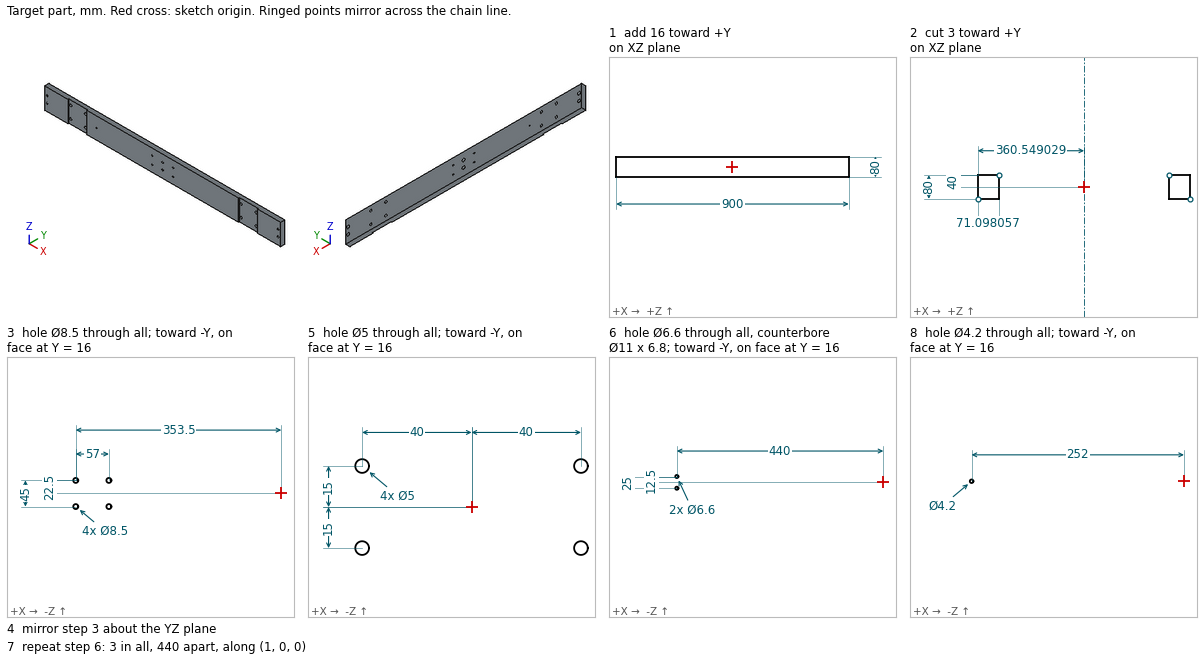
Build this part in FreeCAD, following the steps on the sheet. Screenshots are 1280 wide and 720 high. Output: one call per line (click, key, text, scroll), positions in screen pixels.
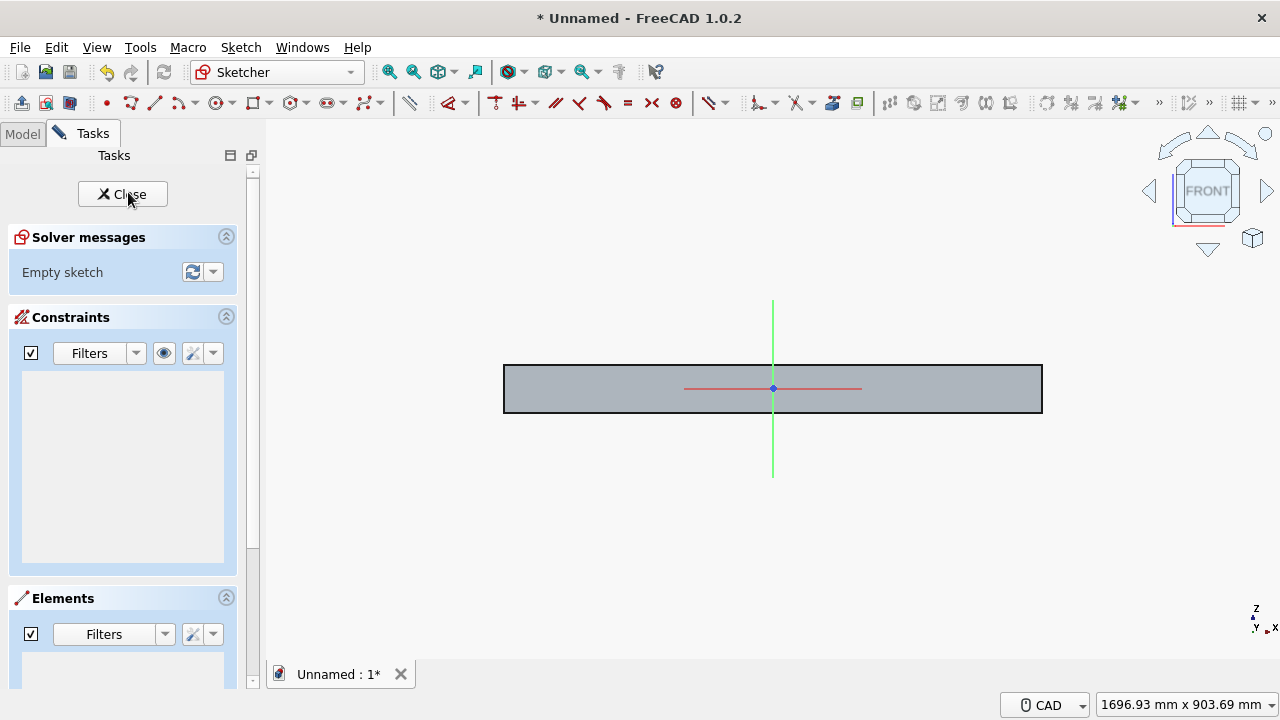
click(254, 104)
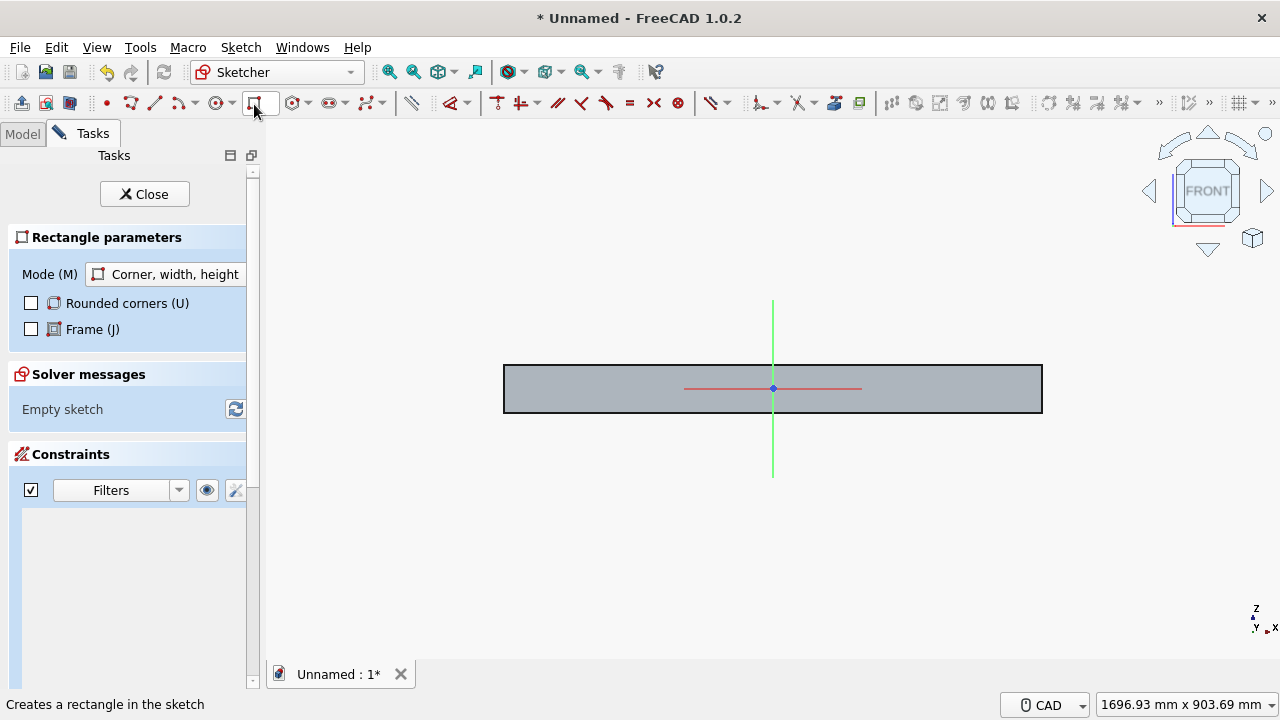
click(558, 365)
click(600, 413)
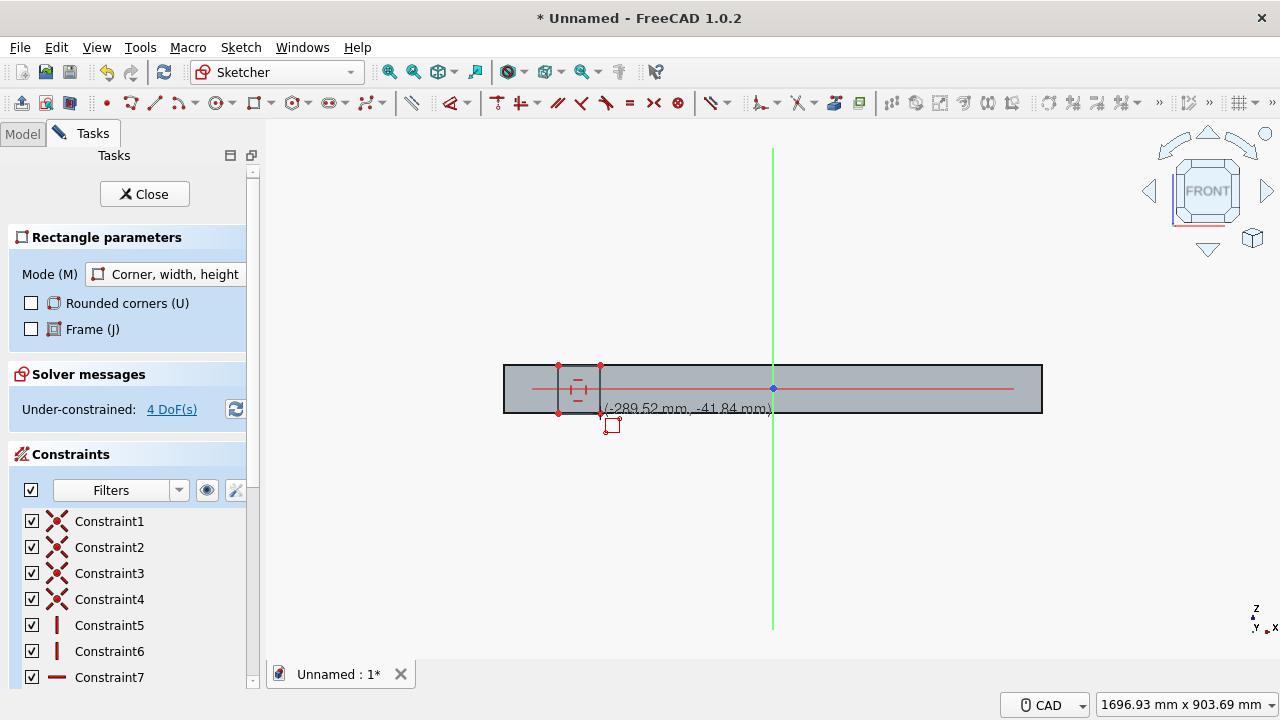
click(946, 365)
click(988, 413)
key(Escape)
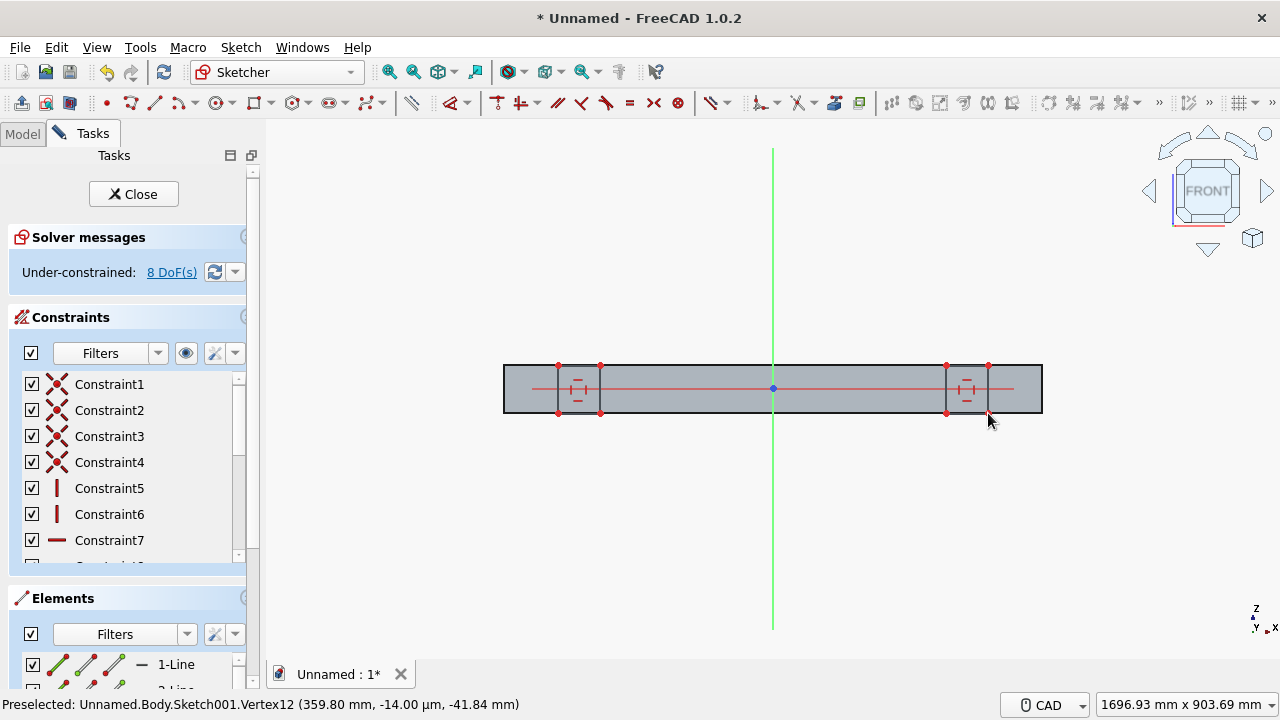
click(600, 366)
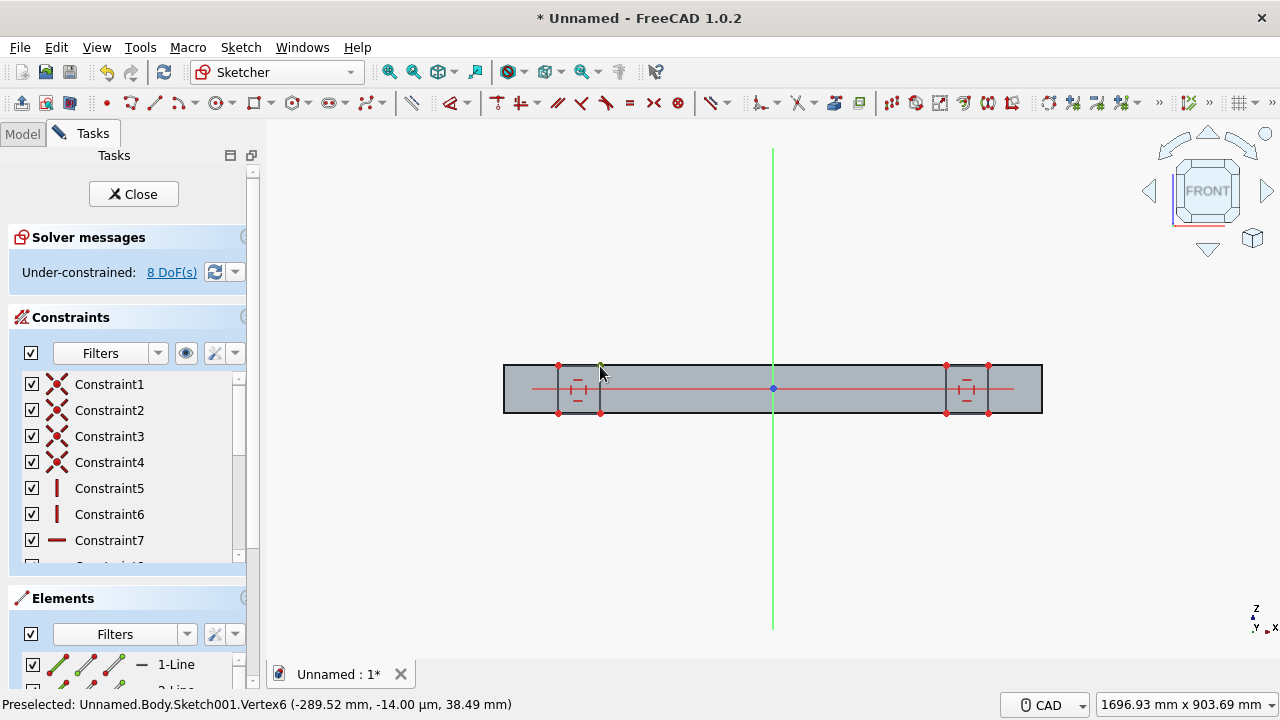
click(946, 366)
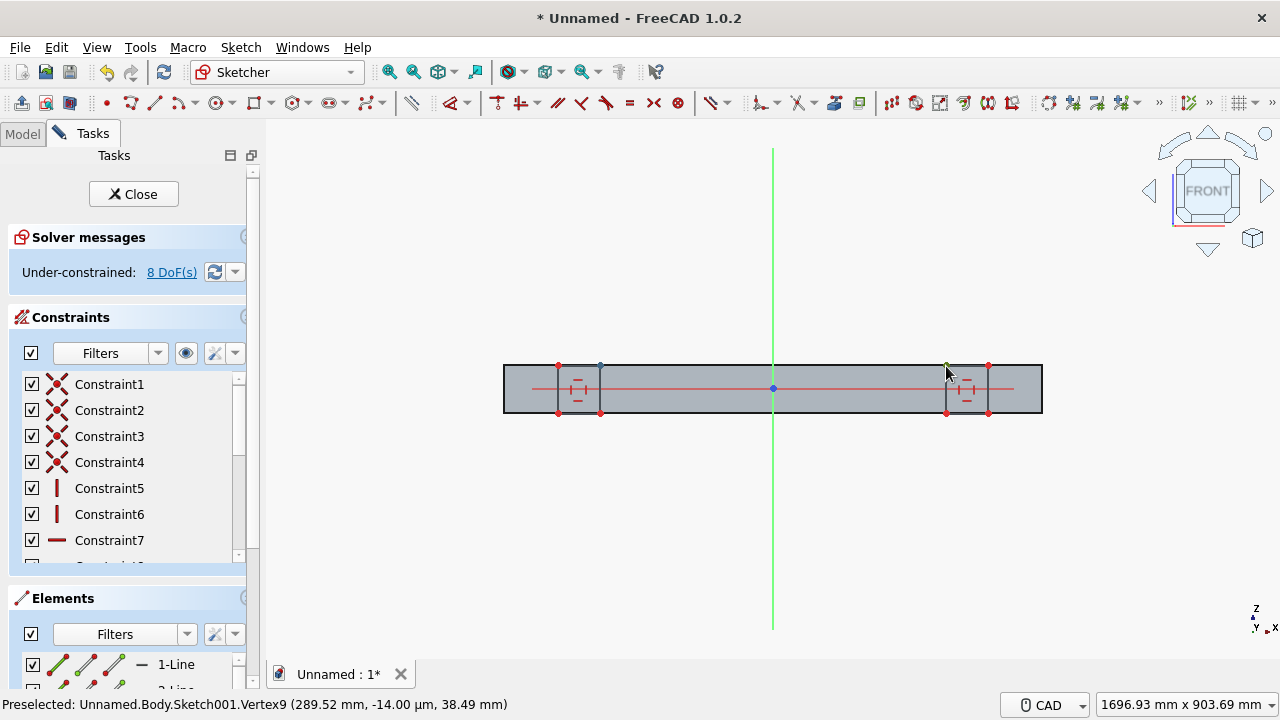
click(773, 596)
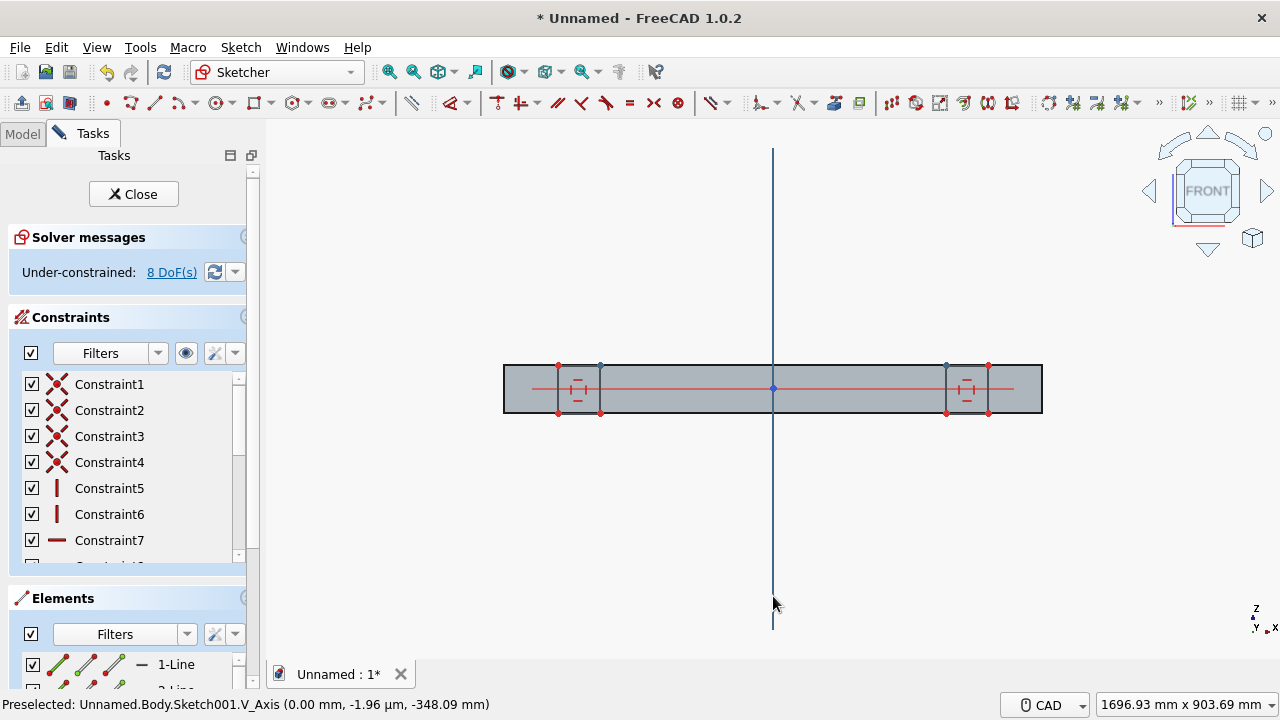
click(654, 104)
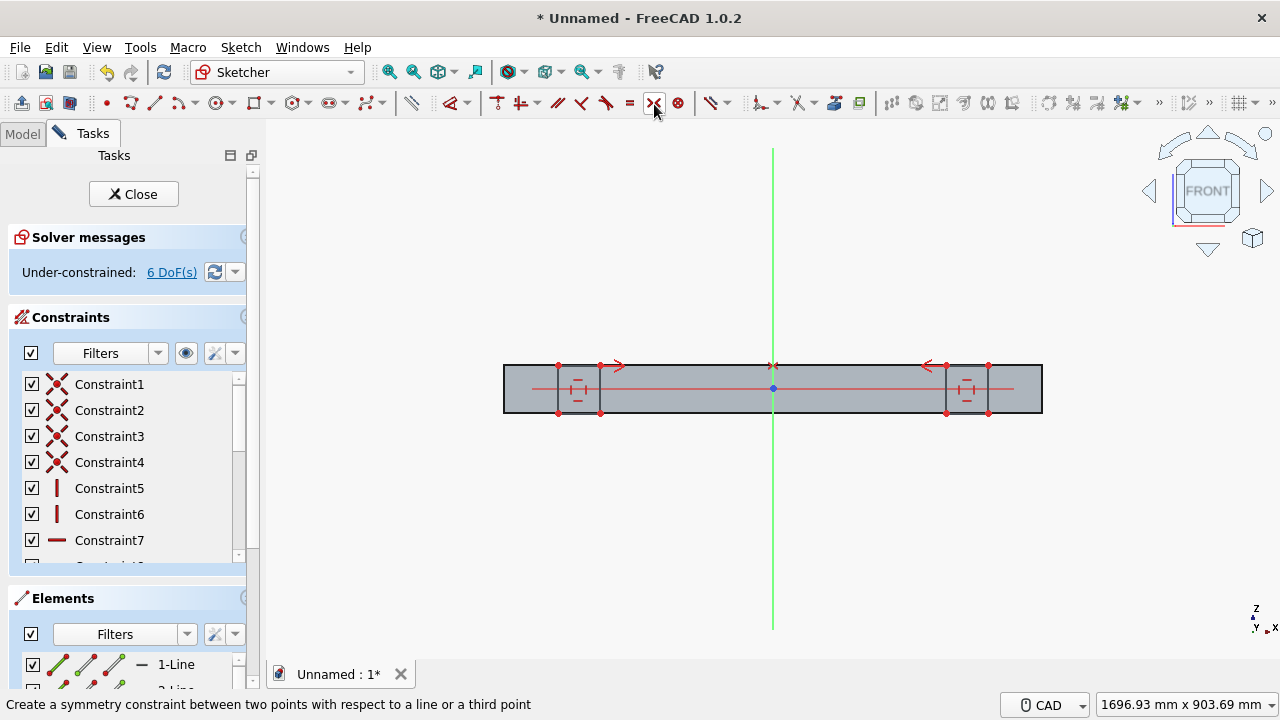
click(558, 414)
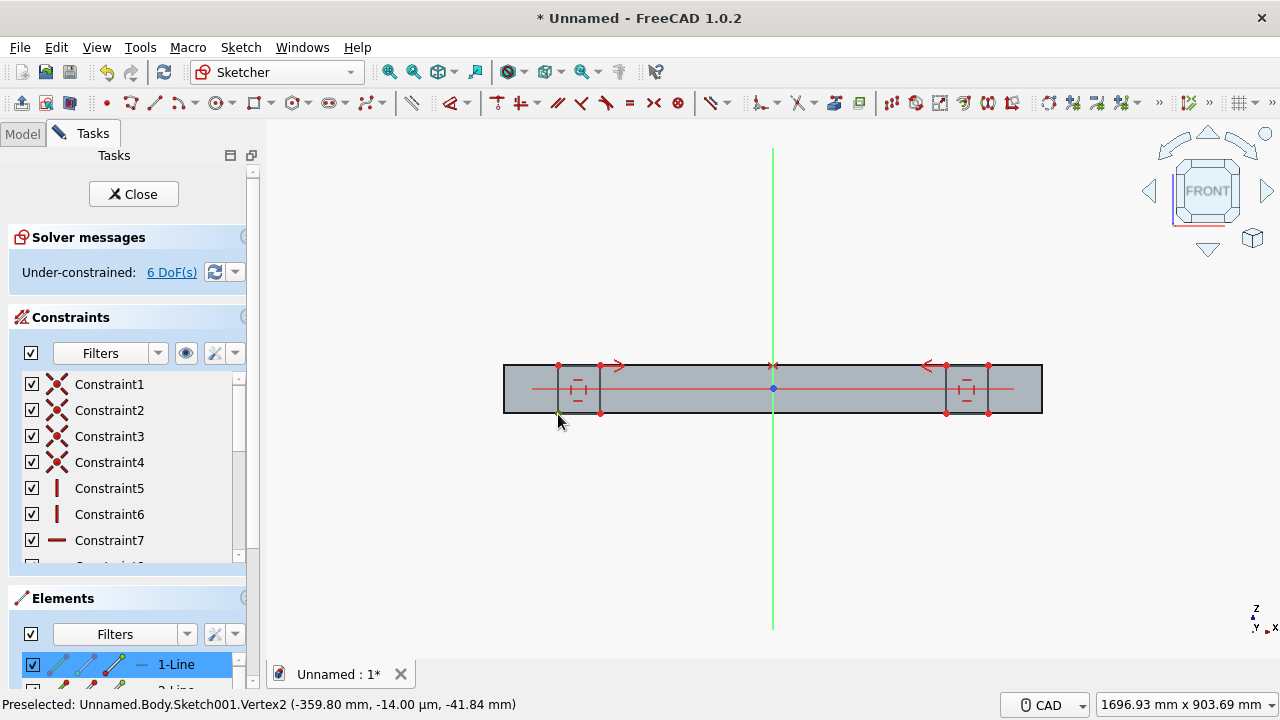
click(988, 414)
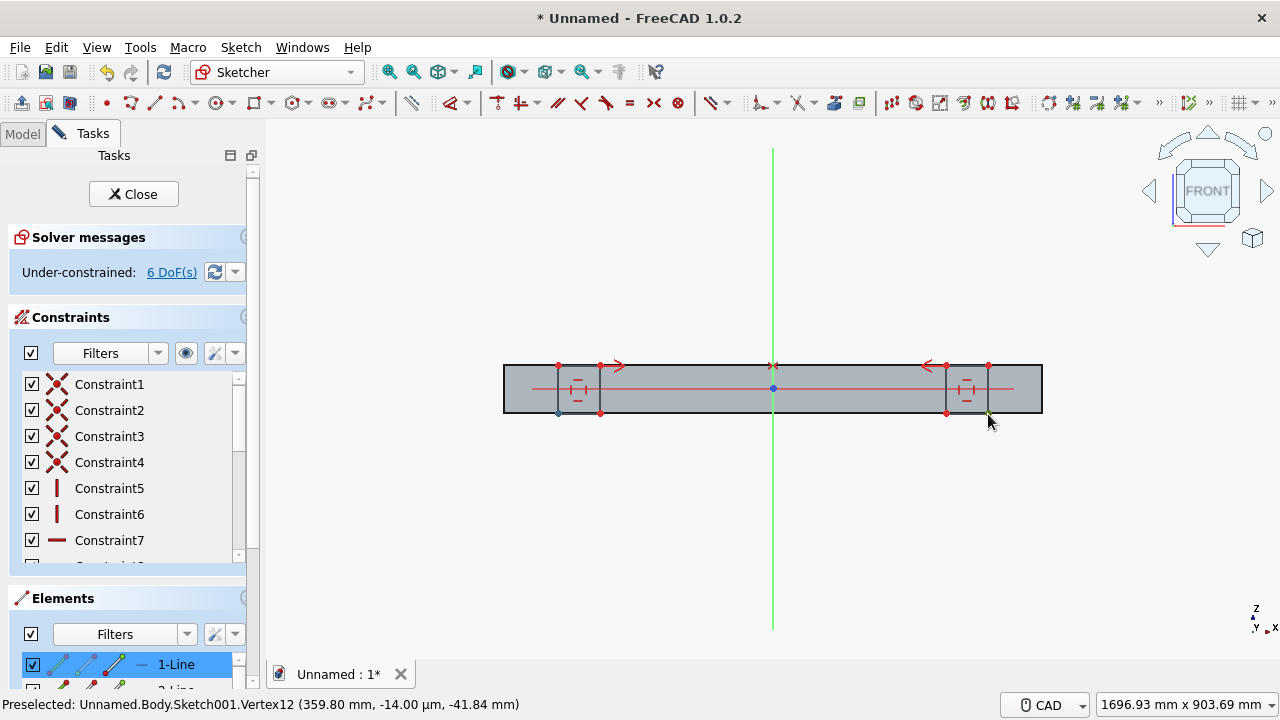
click(773, 596)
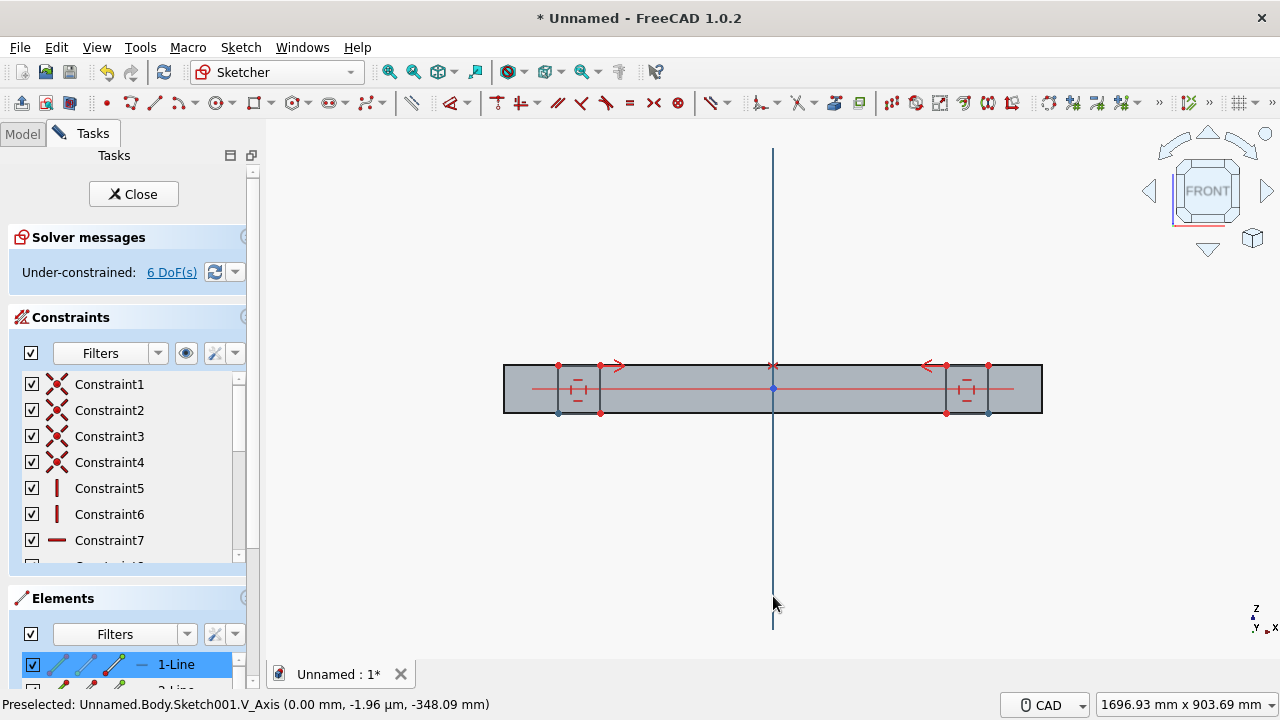
click(654, 104)